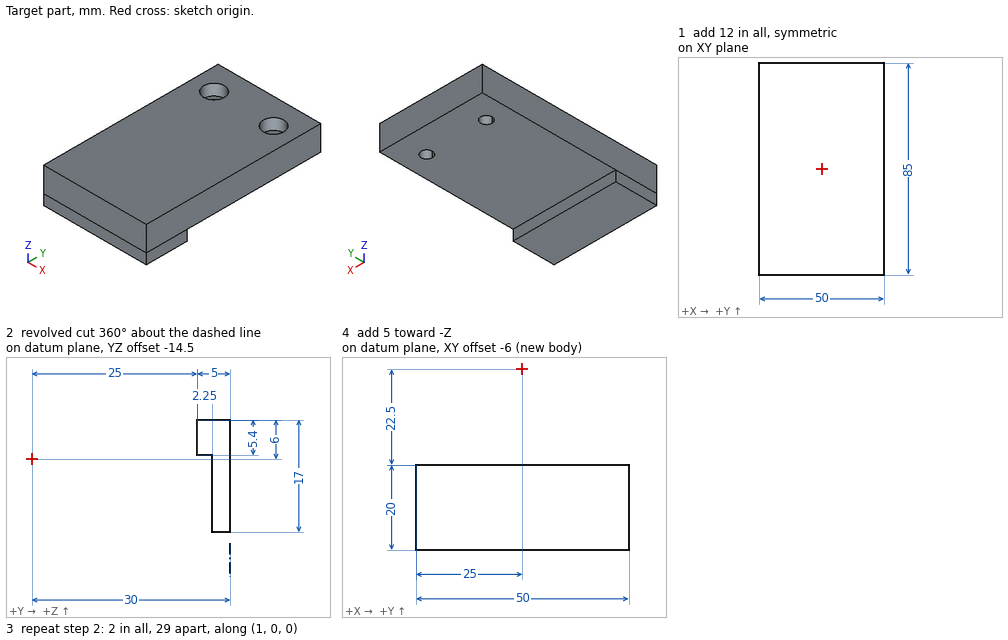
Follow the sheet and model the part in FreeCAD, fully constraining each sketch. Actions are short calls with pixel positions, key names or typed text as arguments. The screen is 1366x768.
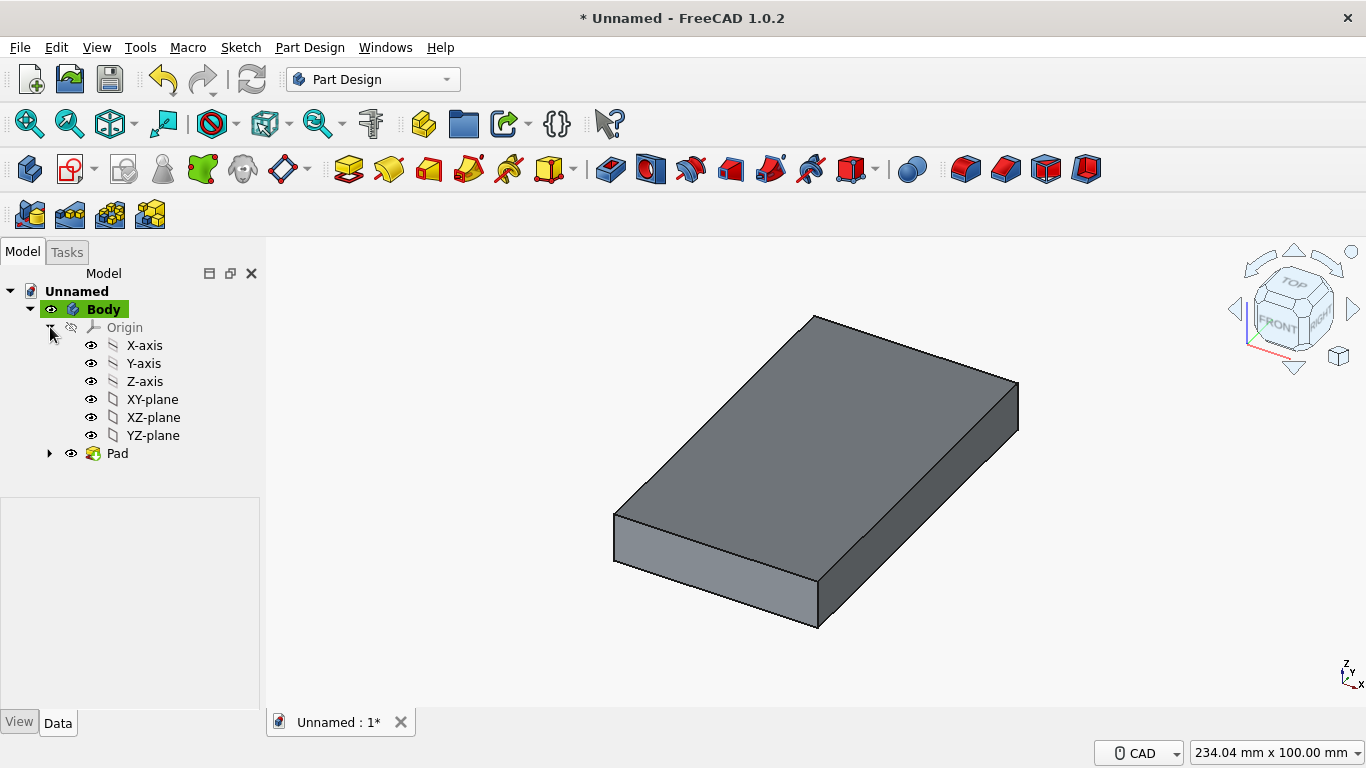
click(136, 435)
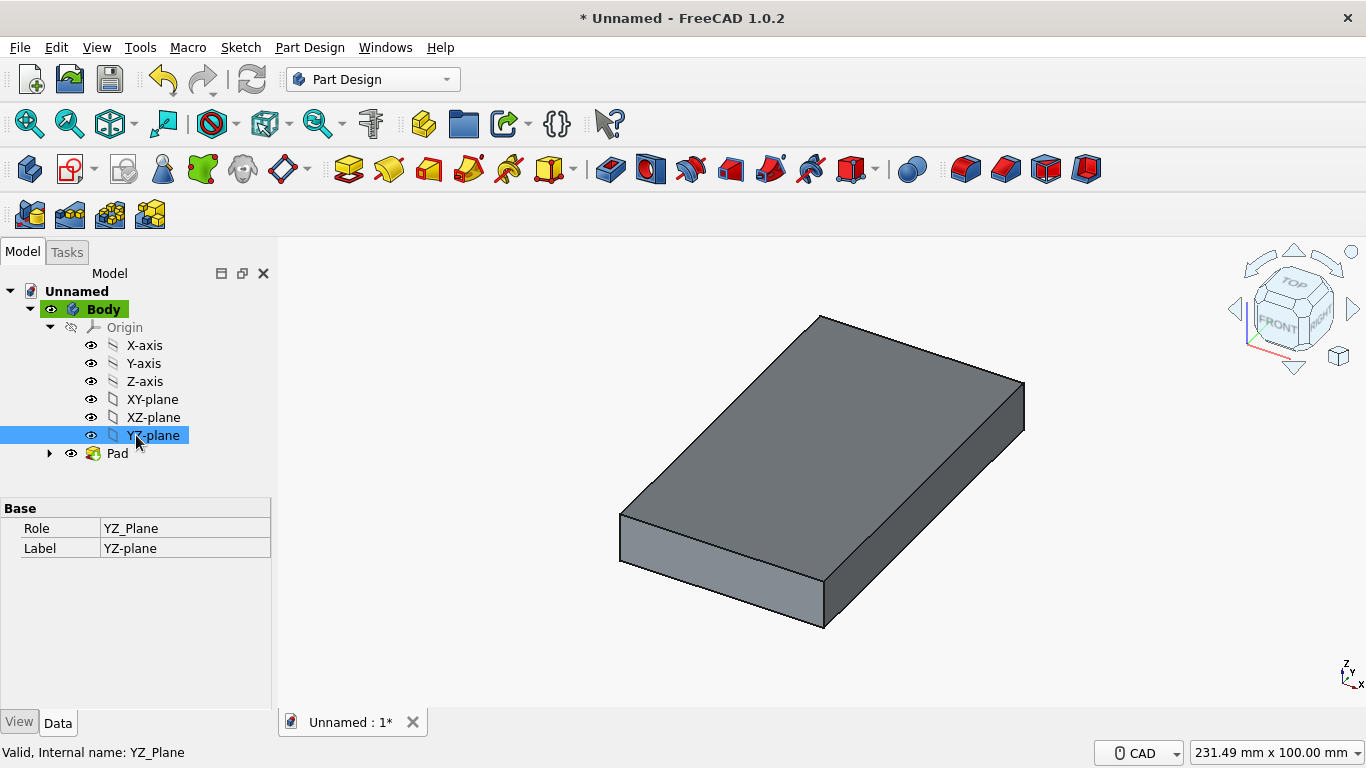
click(284, 170)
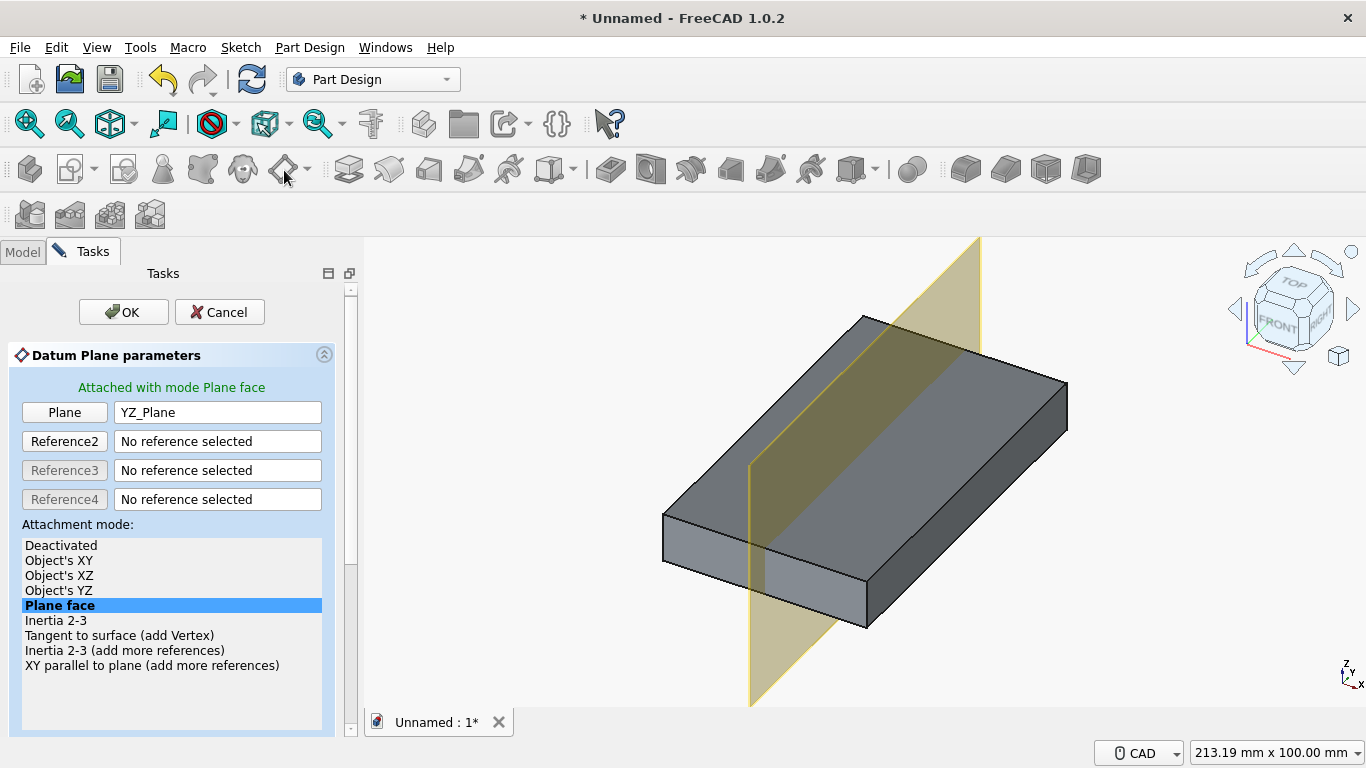
scroll(351, 510, down, 3)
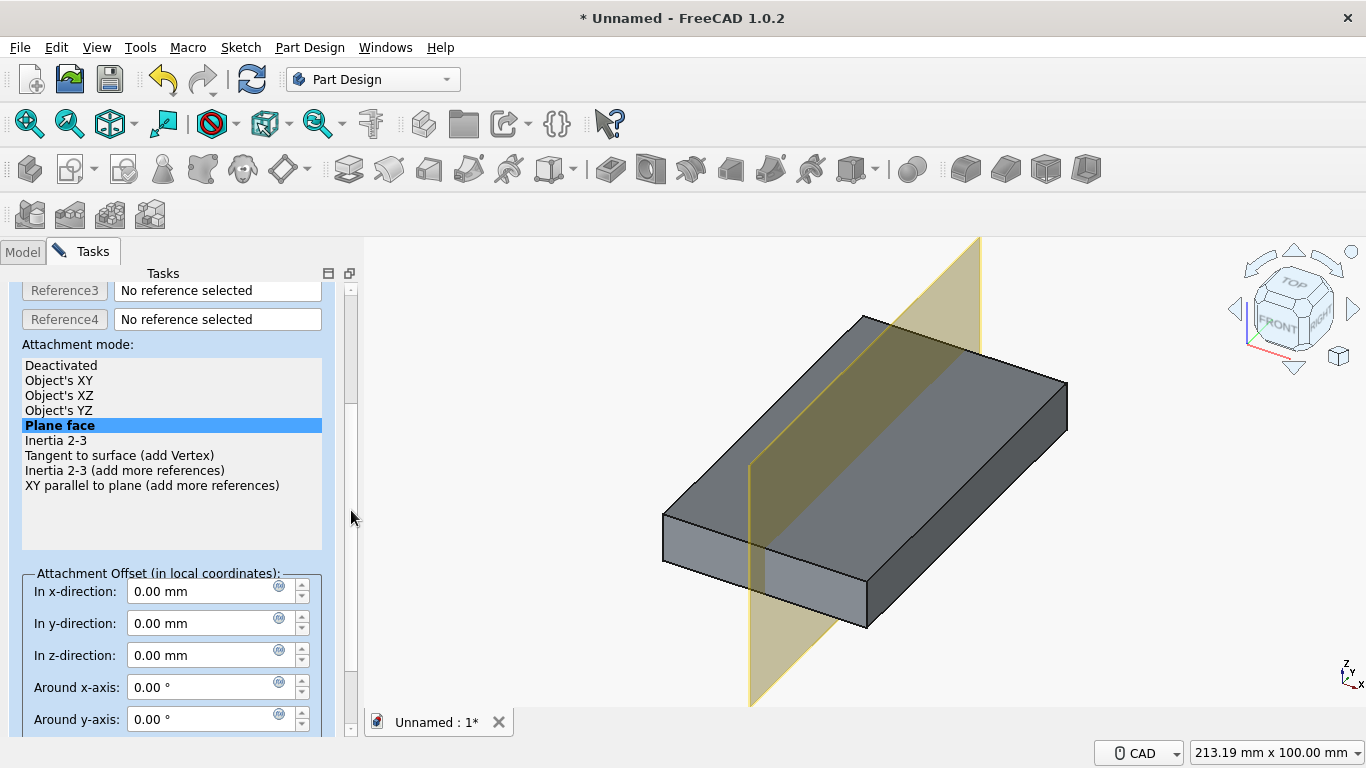
triple_click(210, 655)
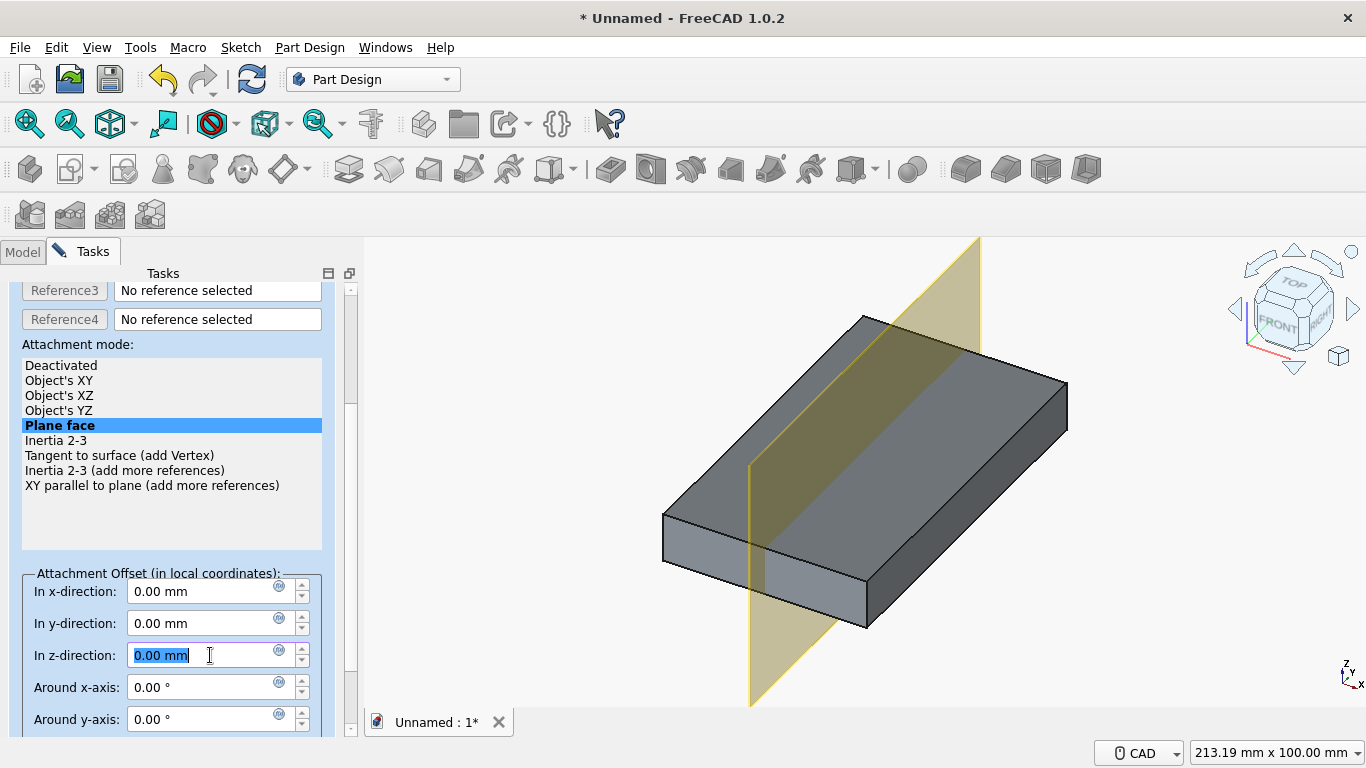
text(-14.5)
key(Tab)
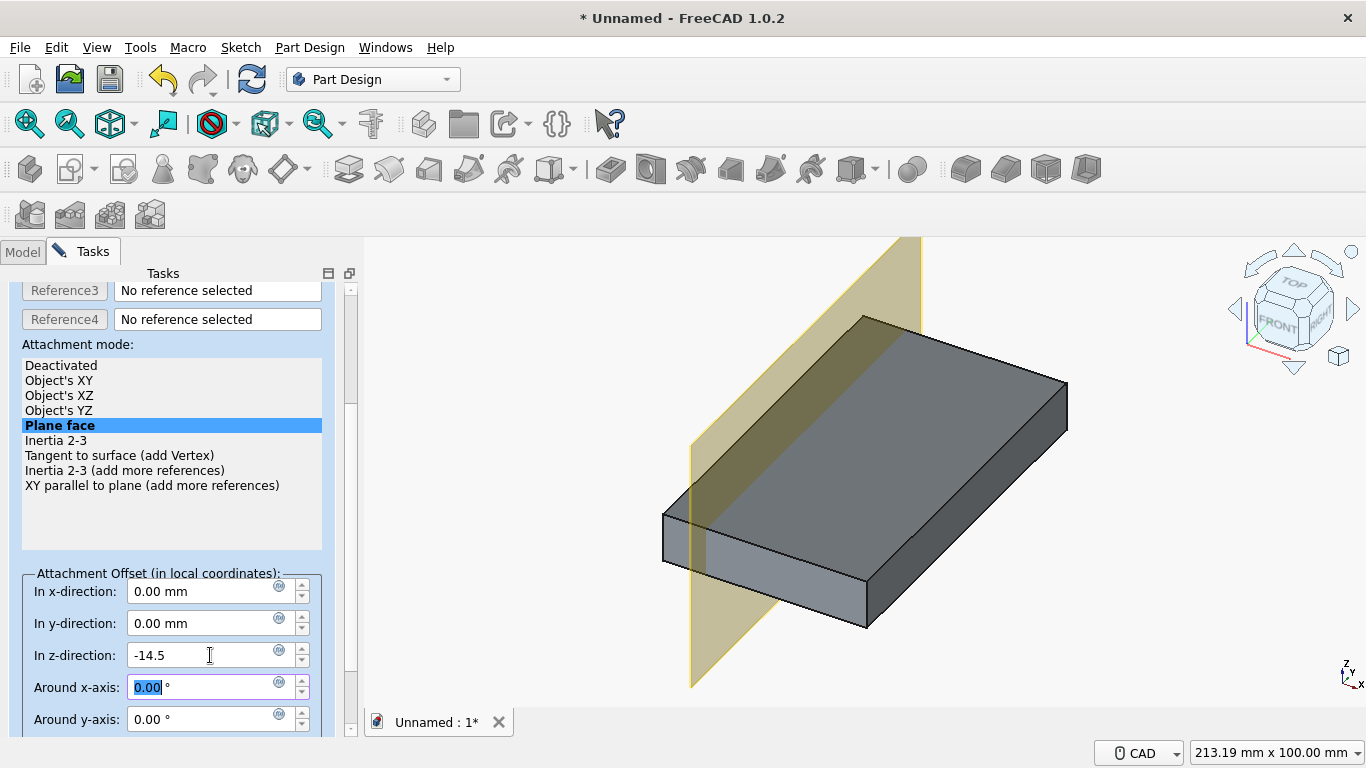
scroll(351, 510, up, 4)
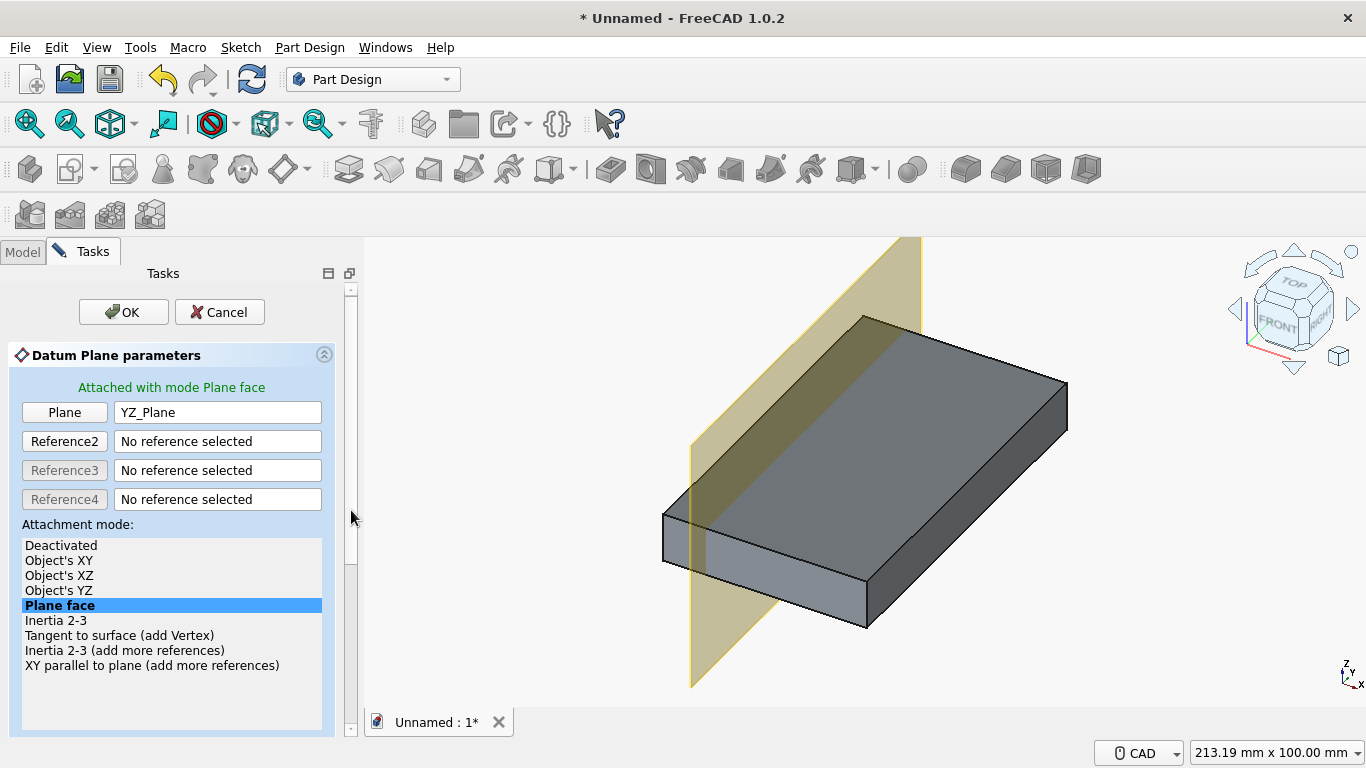
click(124, 312)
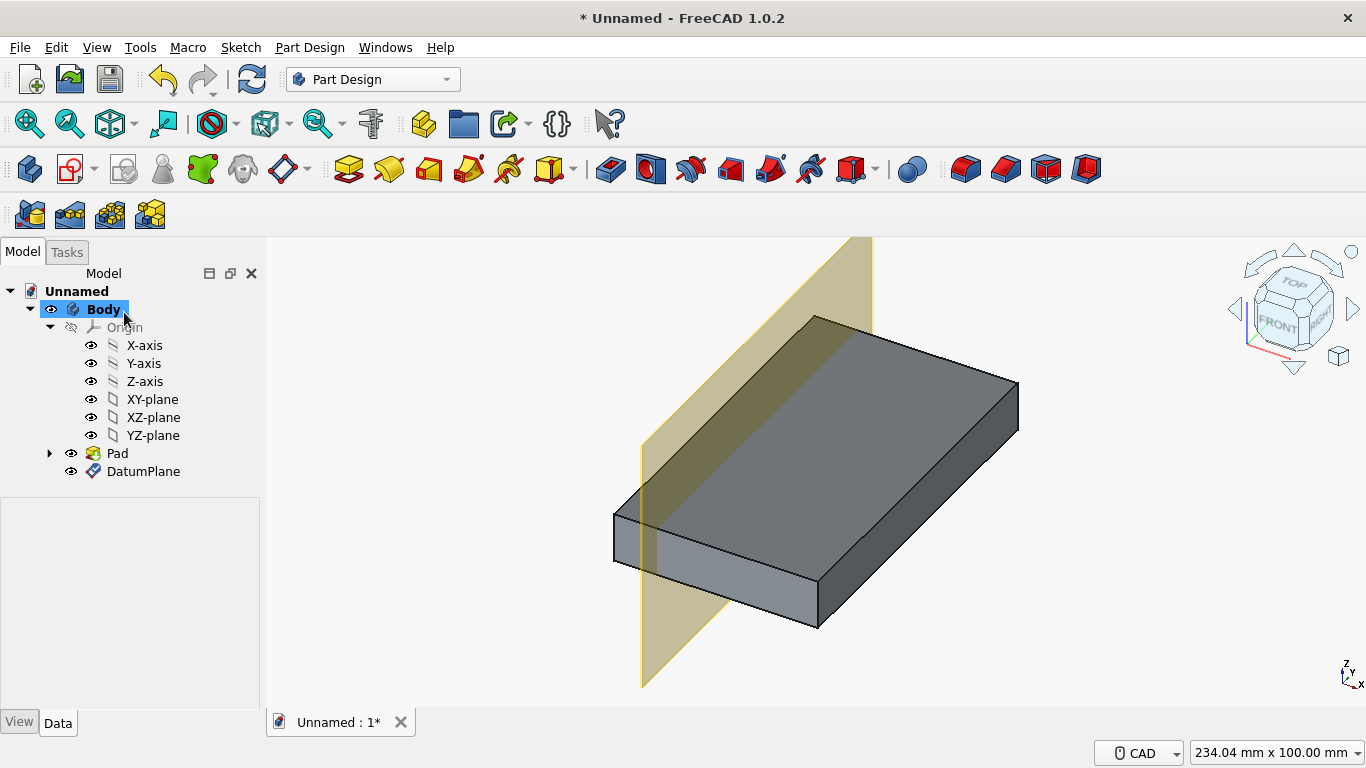
click(116, 471)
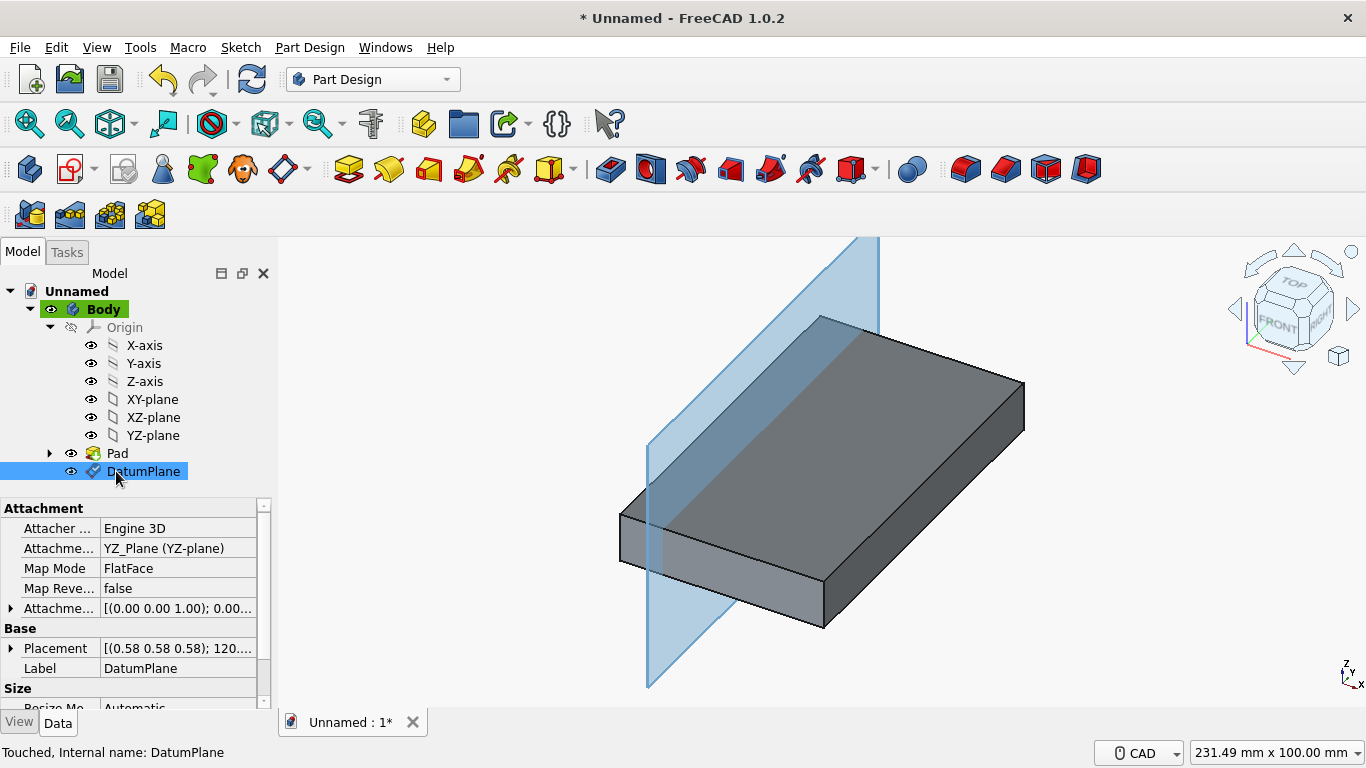
click(70, 170)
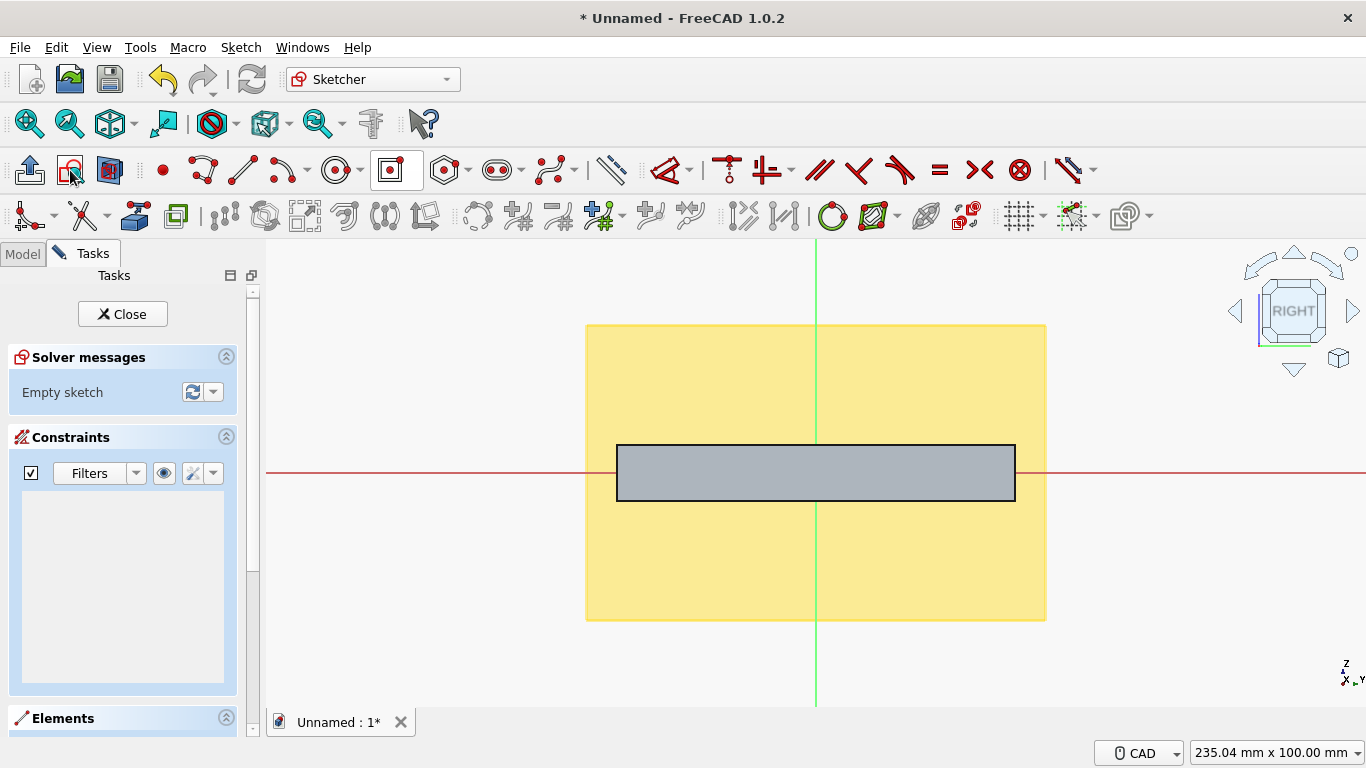
key(q)
key(s)